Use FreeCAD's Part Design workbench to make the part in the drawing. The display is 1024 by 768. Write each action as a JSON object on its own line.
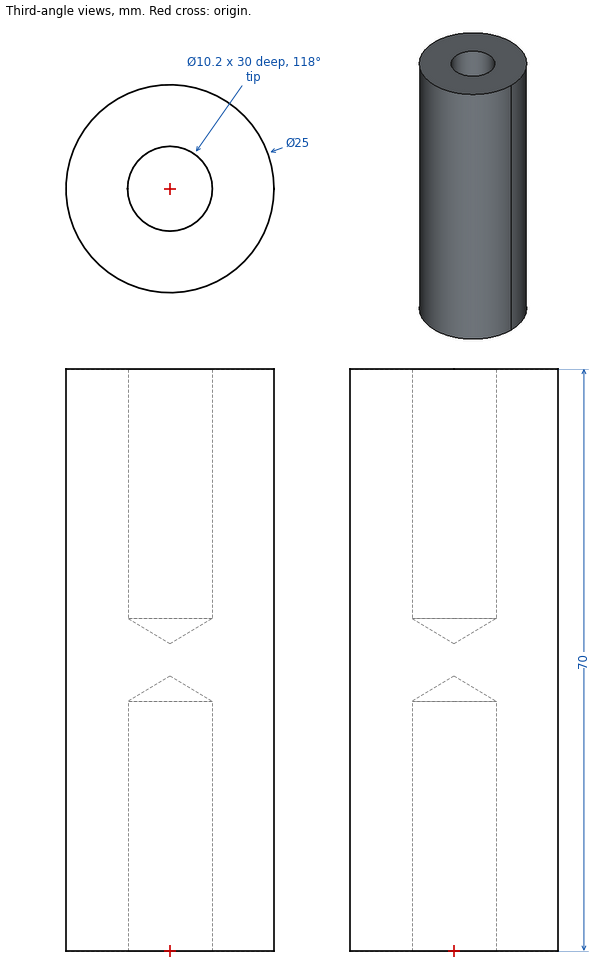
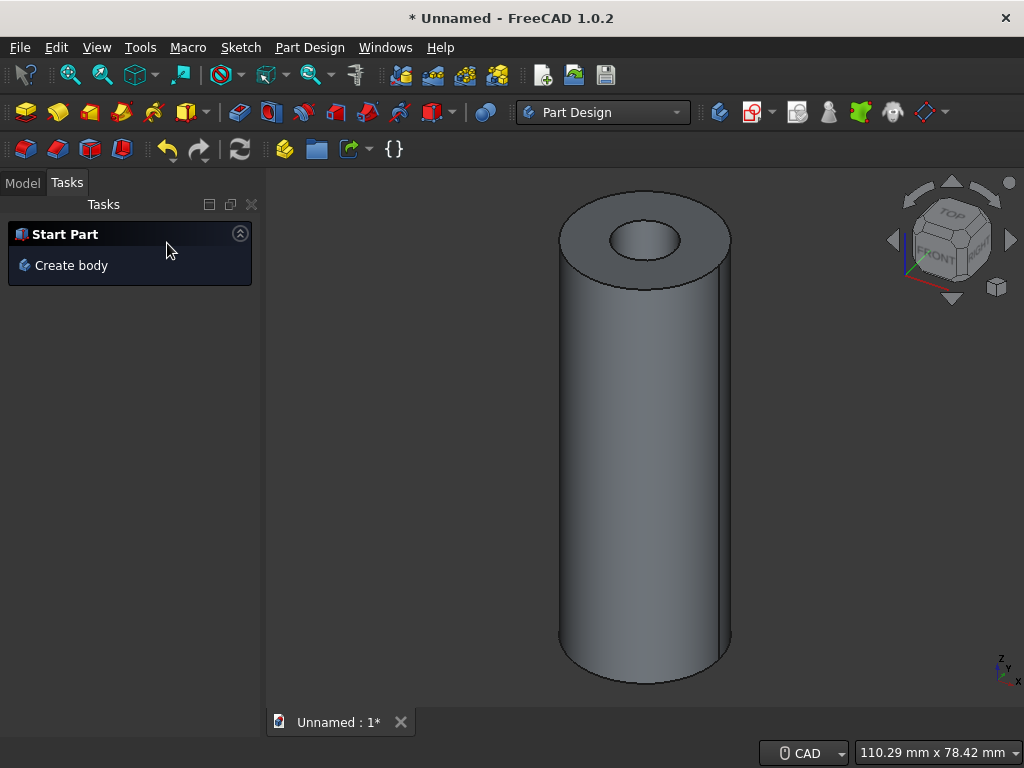
{"action": "key", "text": "5"}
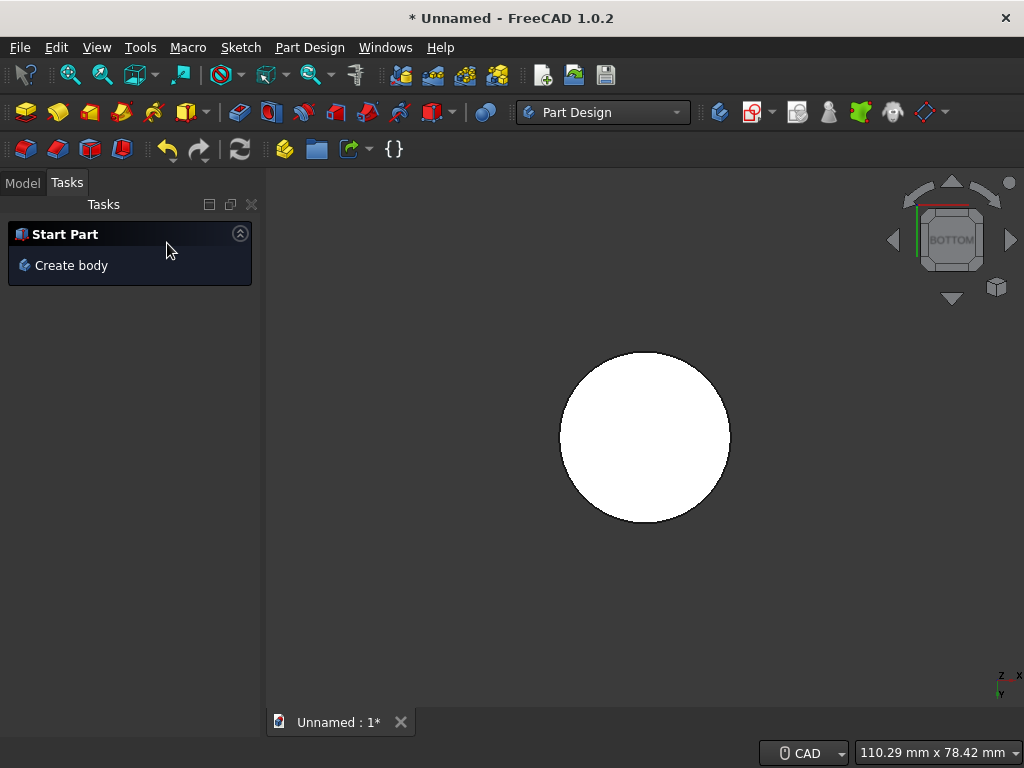
{"action": "key", "text": "v f"}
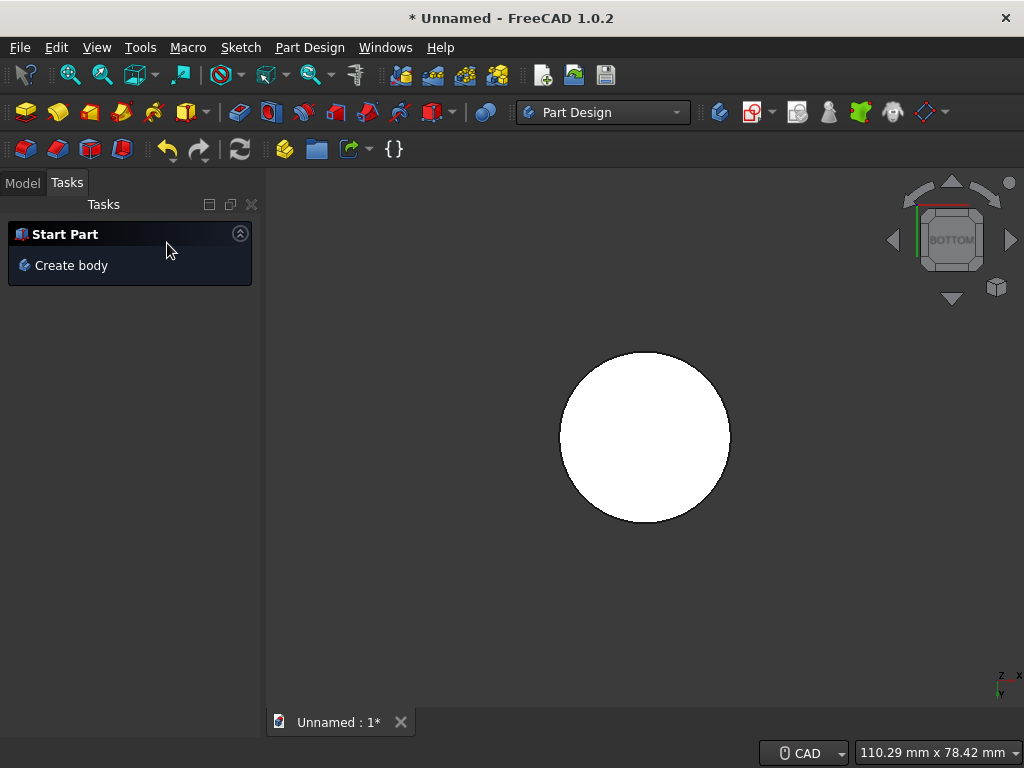
{"action": "left_click", "coordinate": [645, 436]}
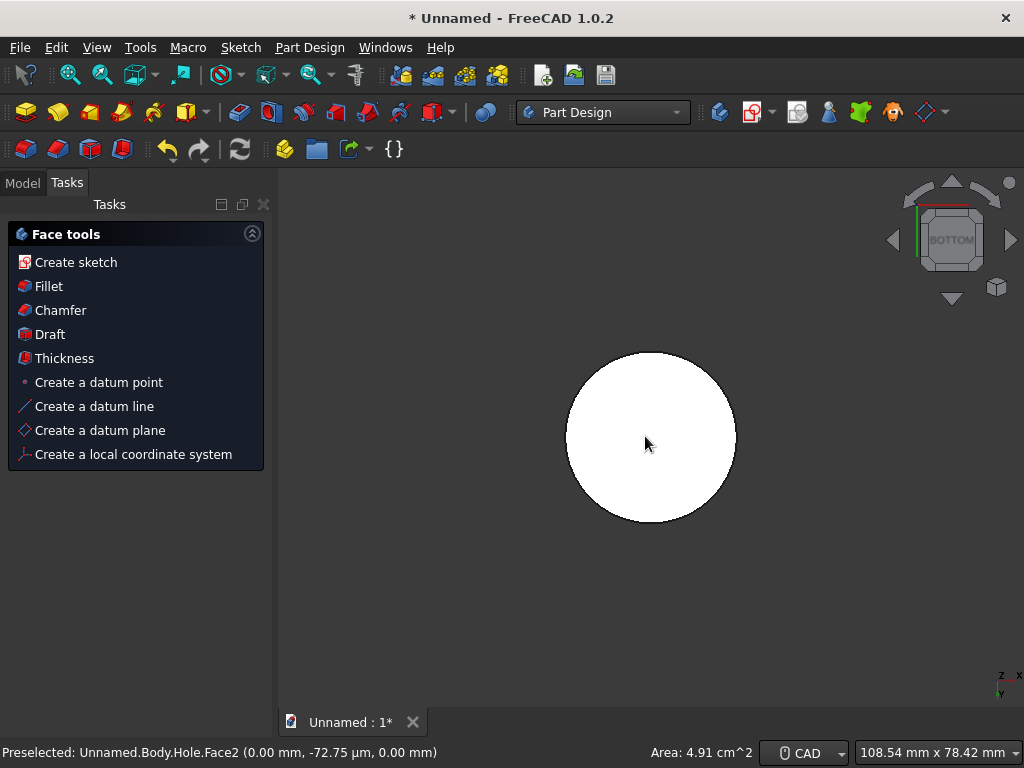
{"action": "left_click", "coordinate": [752, 112]}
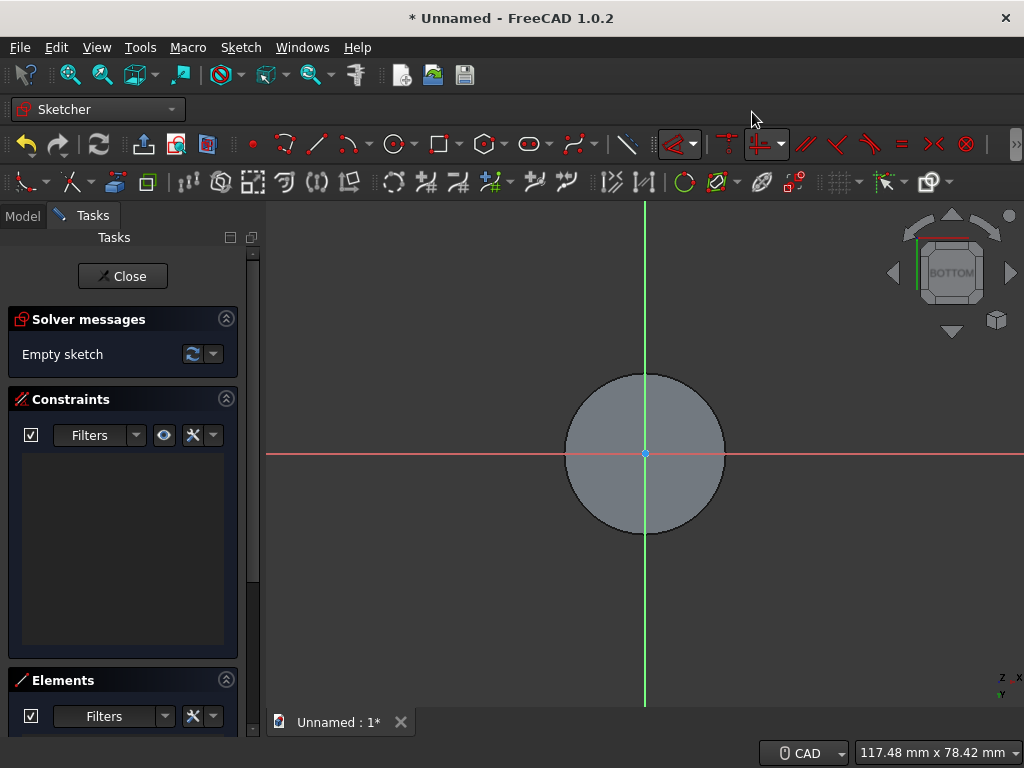
{"action": "scroll", "coordinate": [662, 454], "scroll_direction": "up", "scroll_amount": 8}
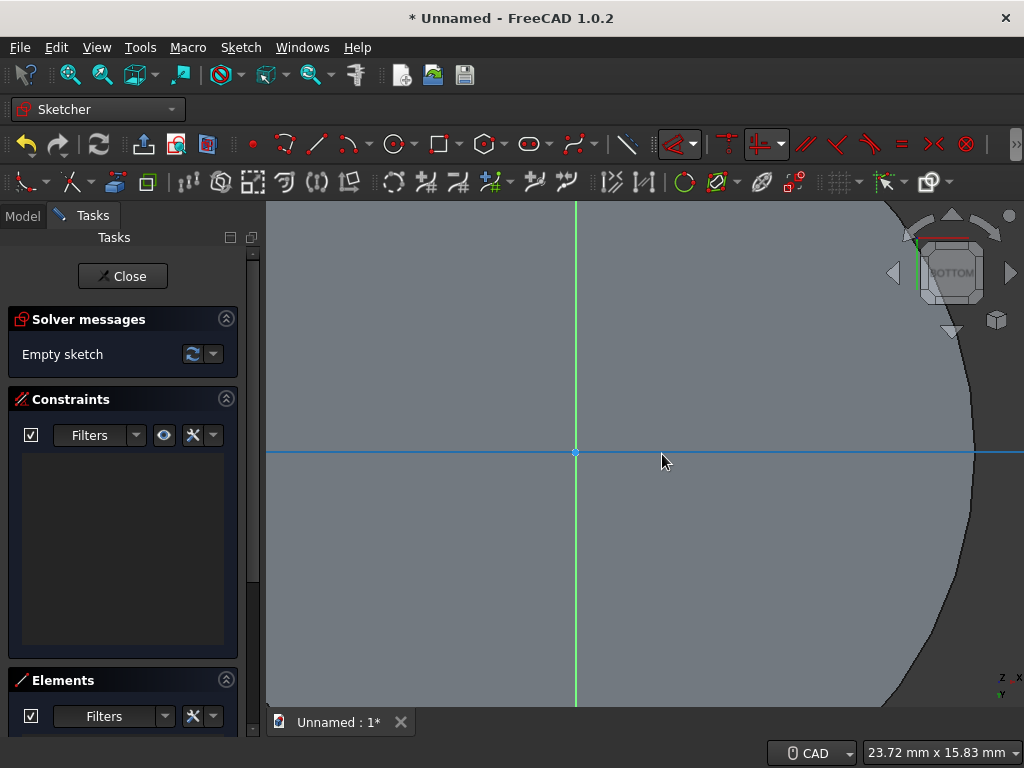
{"action": "left_click", "coordinate": [394, 144]}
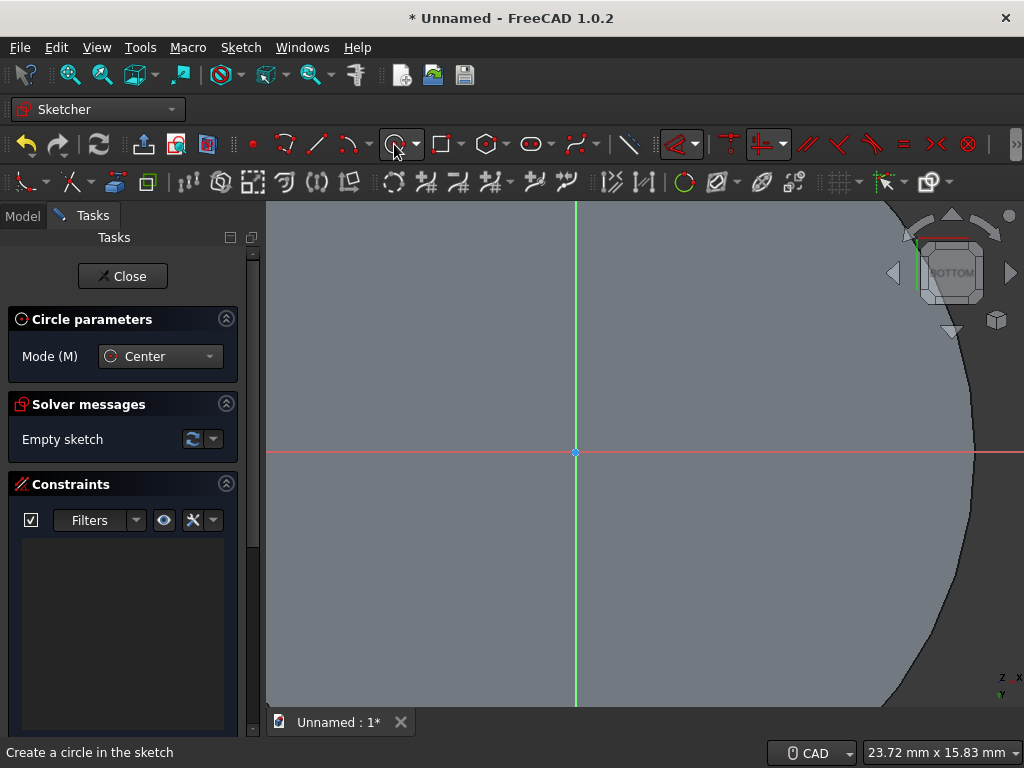
{"action": "left_click", "coordinate": [576, 452]}
{"action": "mouse_move", "coordinate": [691, 337]}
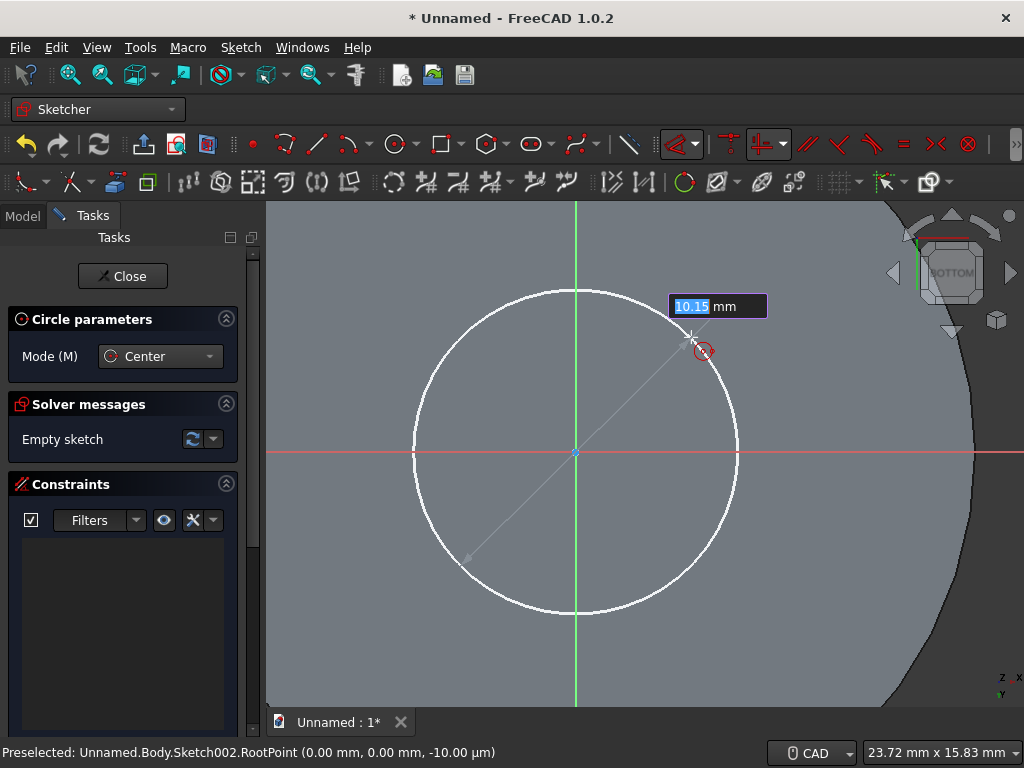
{"action": "type", "text": "10.2"}
{"action": "key", "text": "Return"}
{"action": "key", "text": "Escape"}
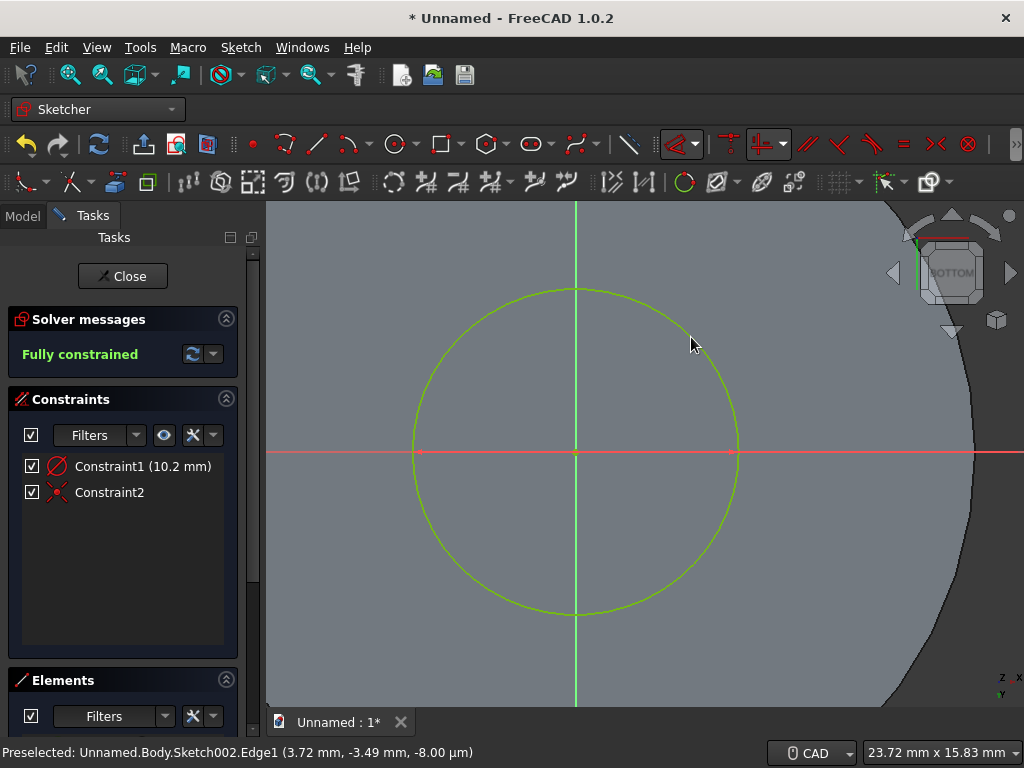
{"action": "left_click", "coordinate": [123, 276]}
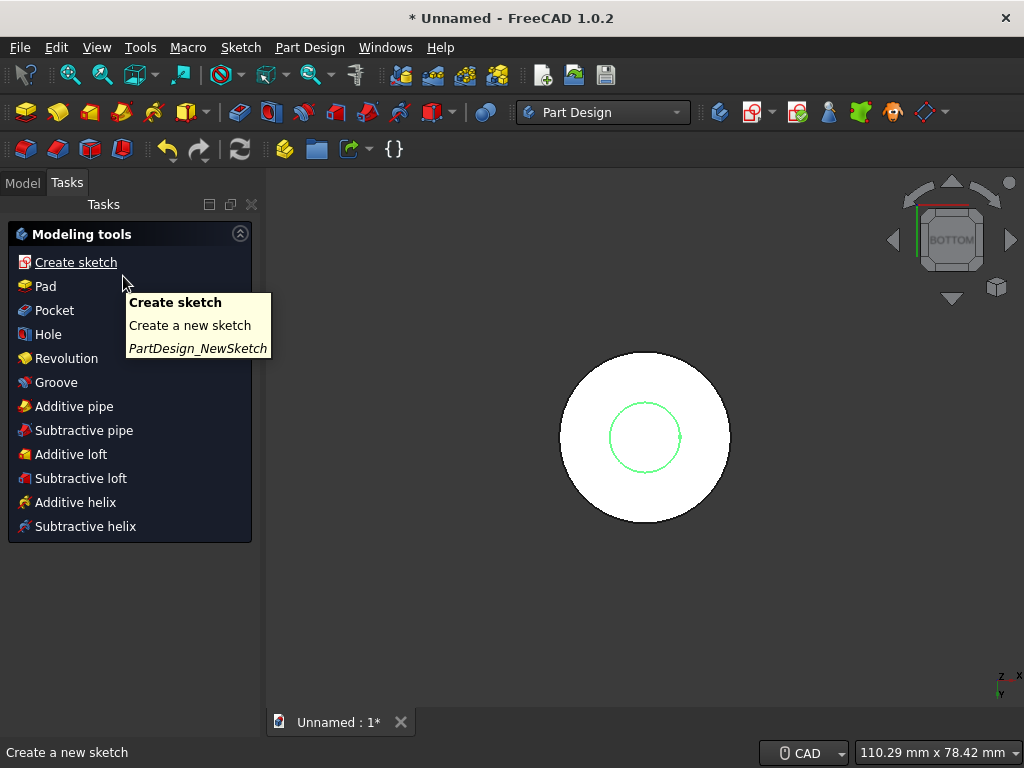
{"action": "left_click", "coordinate": [272, 112]}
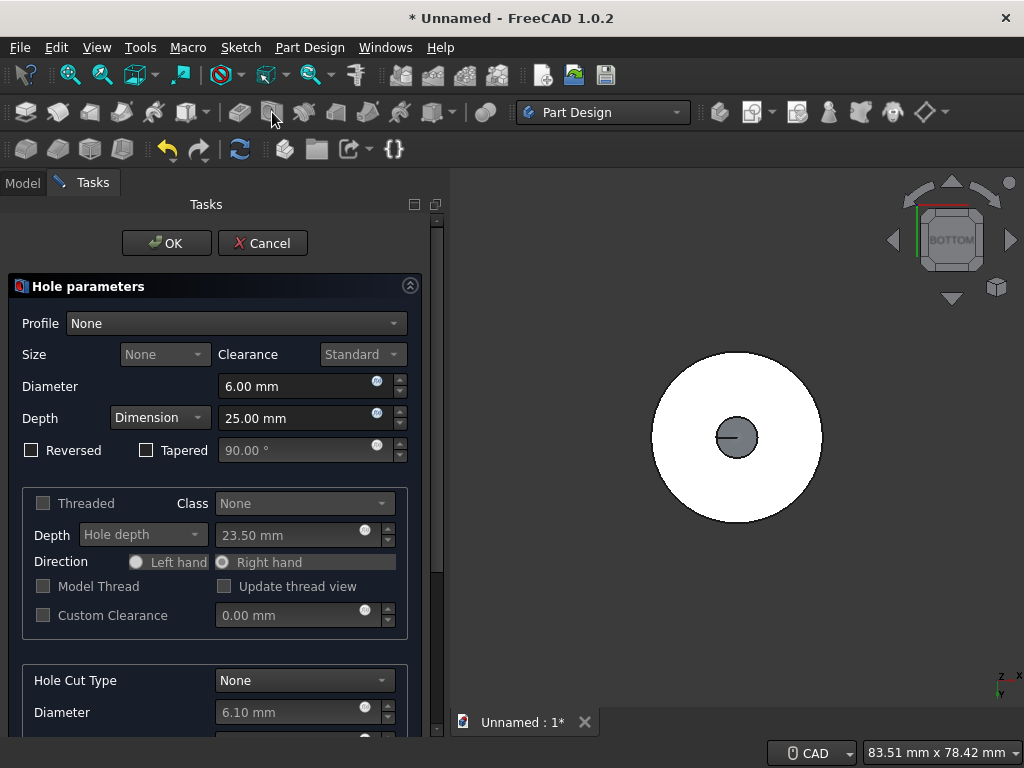
{"action": "triple_click", "coordinate": [305, 386]}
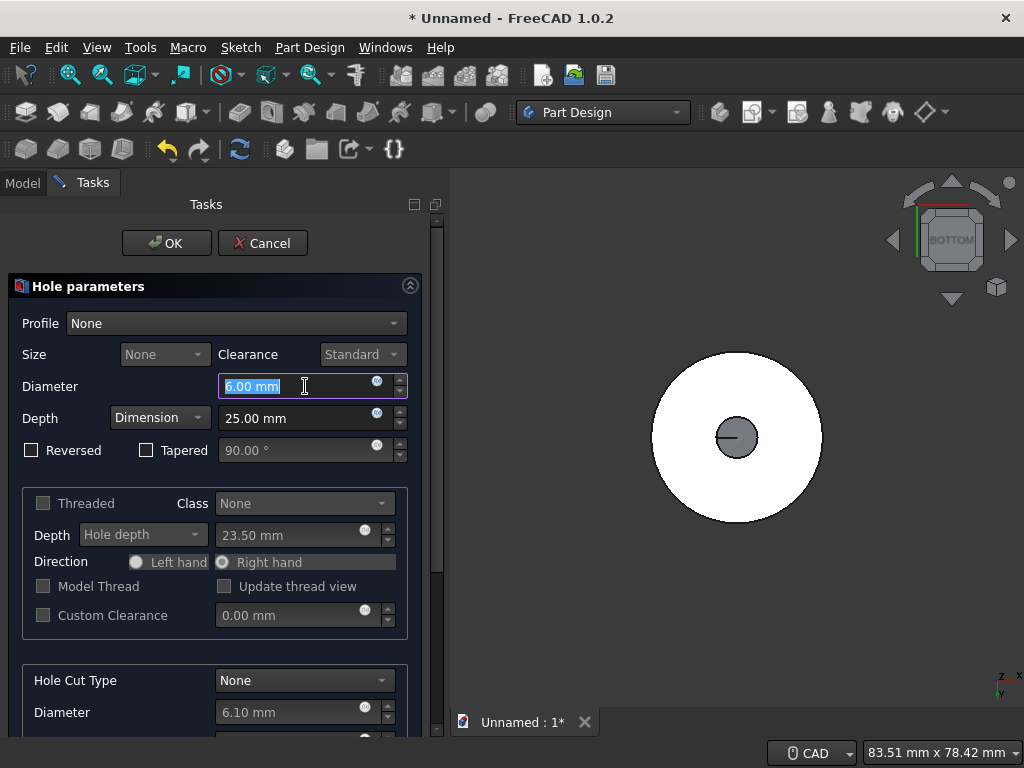
{"action": "type", "text": "10.2"}
{"action": "key", "text": "Tab"}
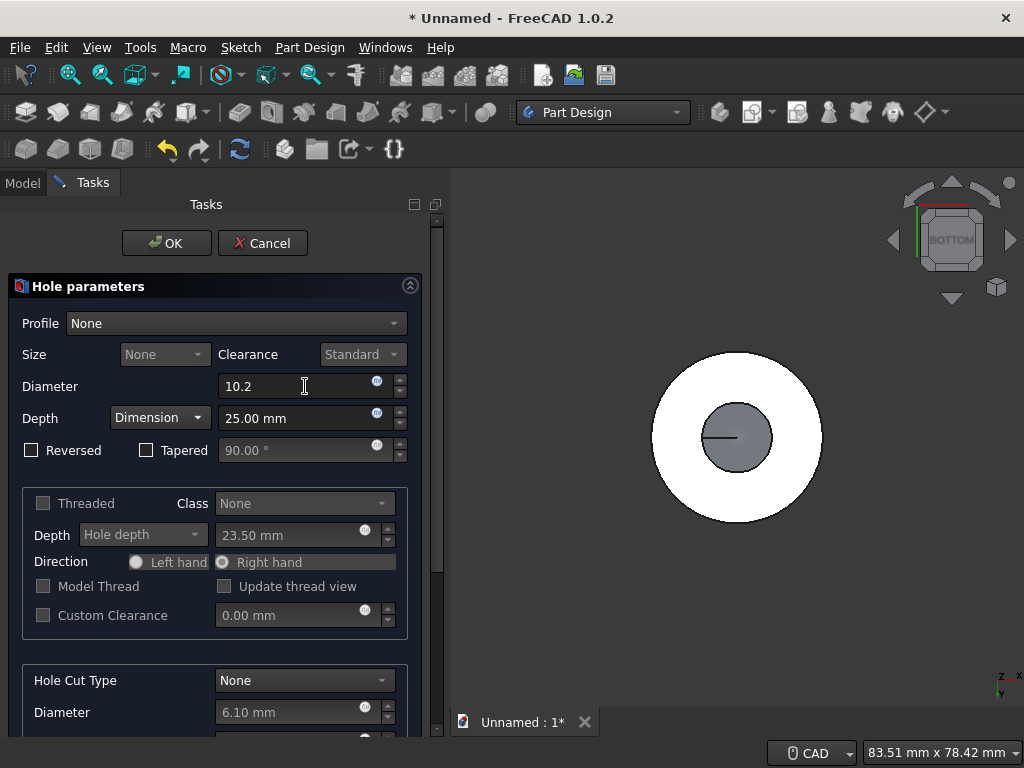
{"action": "triple_click", "coordinate": [305, 418]}